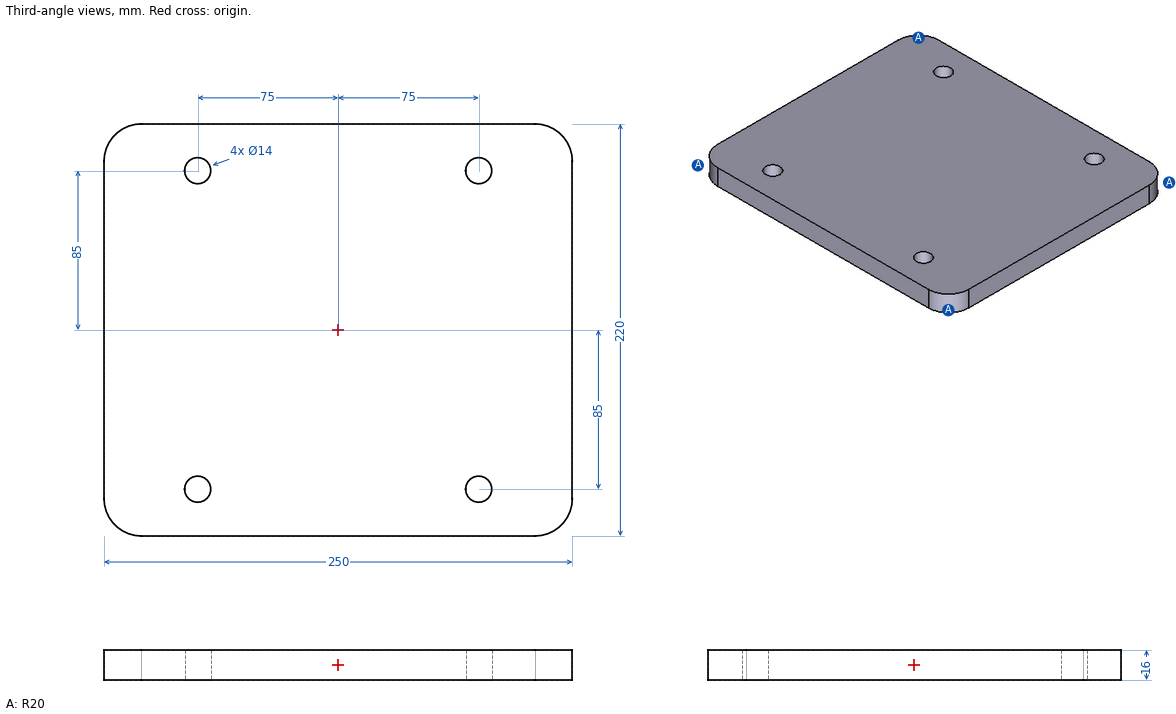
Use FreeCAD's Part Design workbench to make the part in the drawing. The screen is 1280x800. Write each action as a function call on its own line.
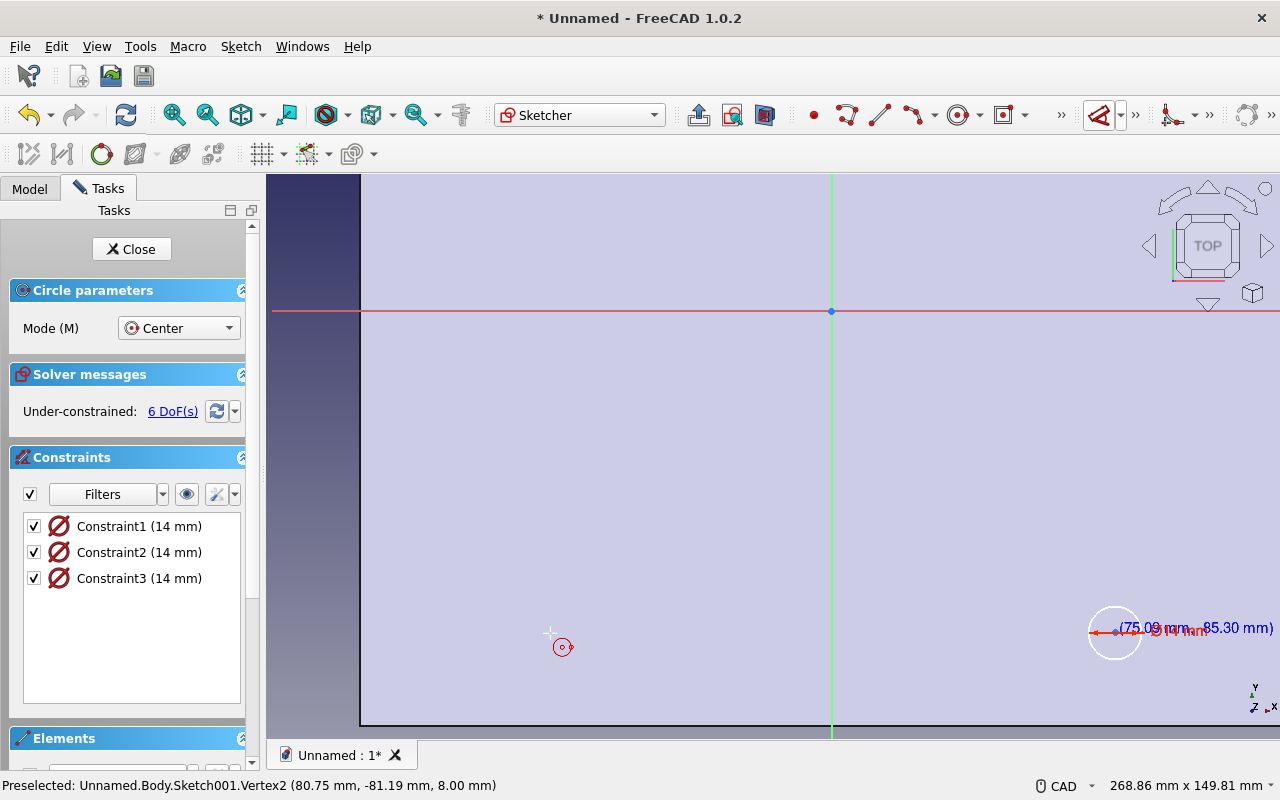
click(549, 632)
move(568, 613)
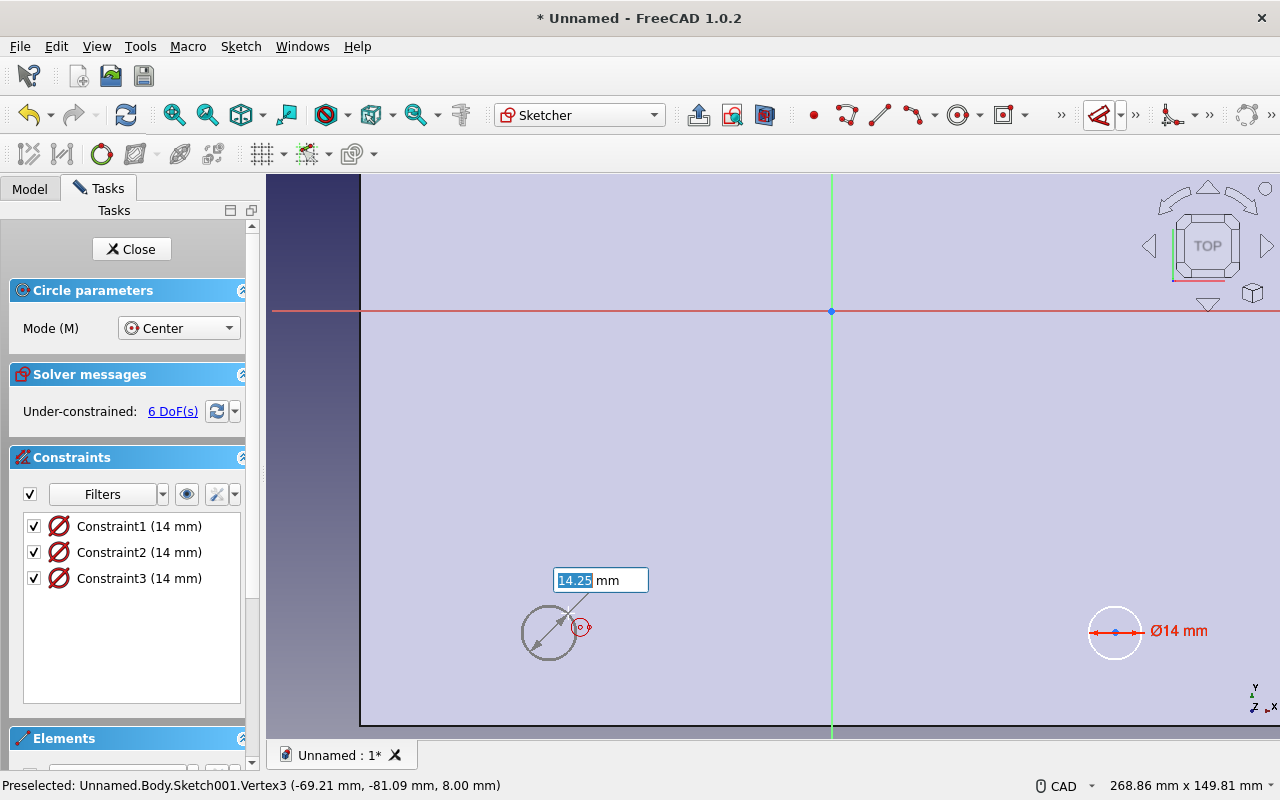
text(14)
key(Return)
key(Escape)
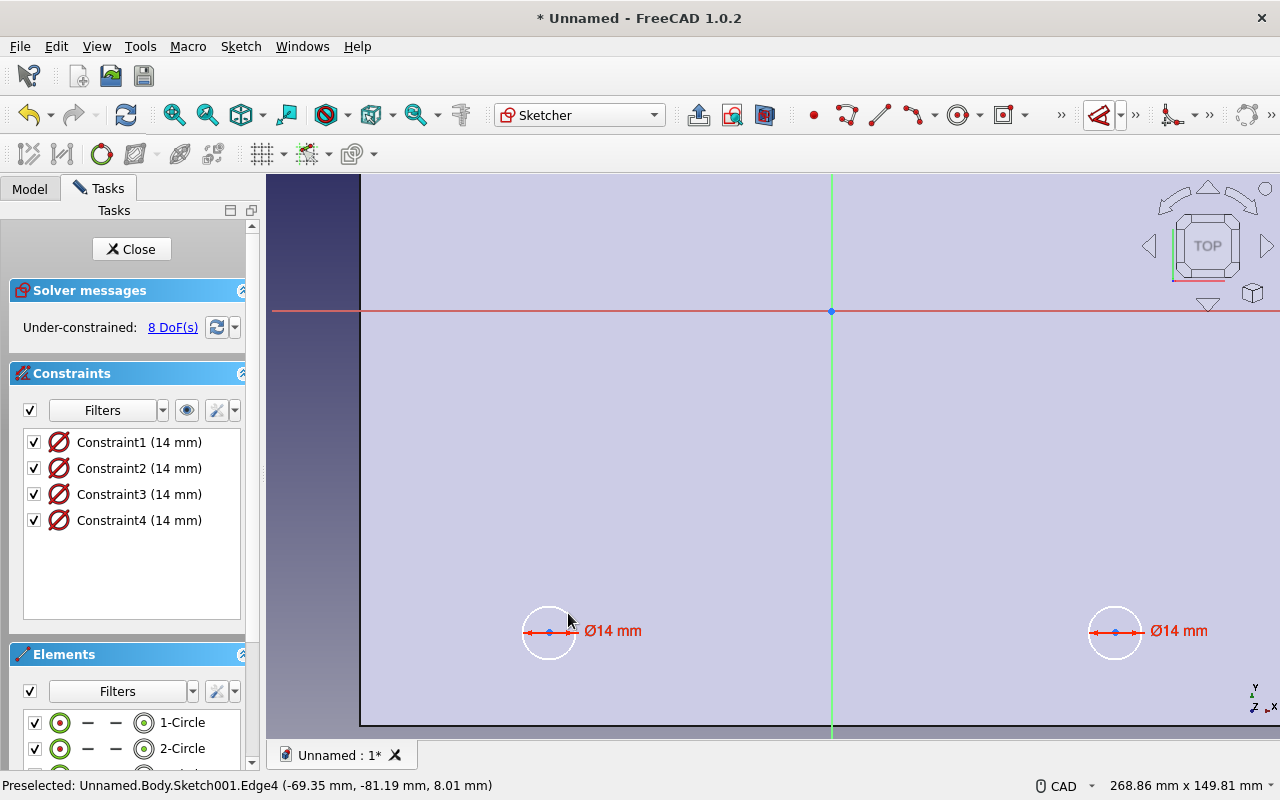
scroll(550, 633, down, 3)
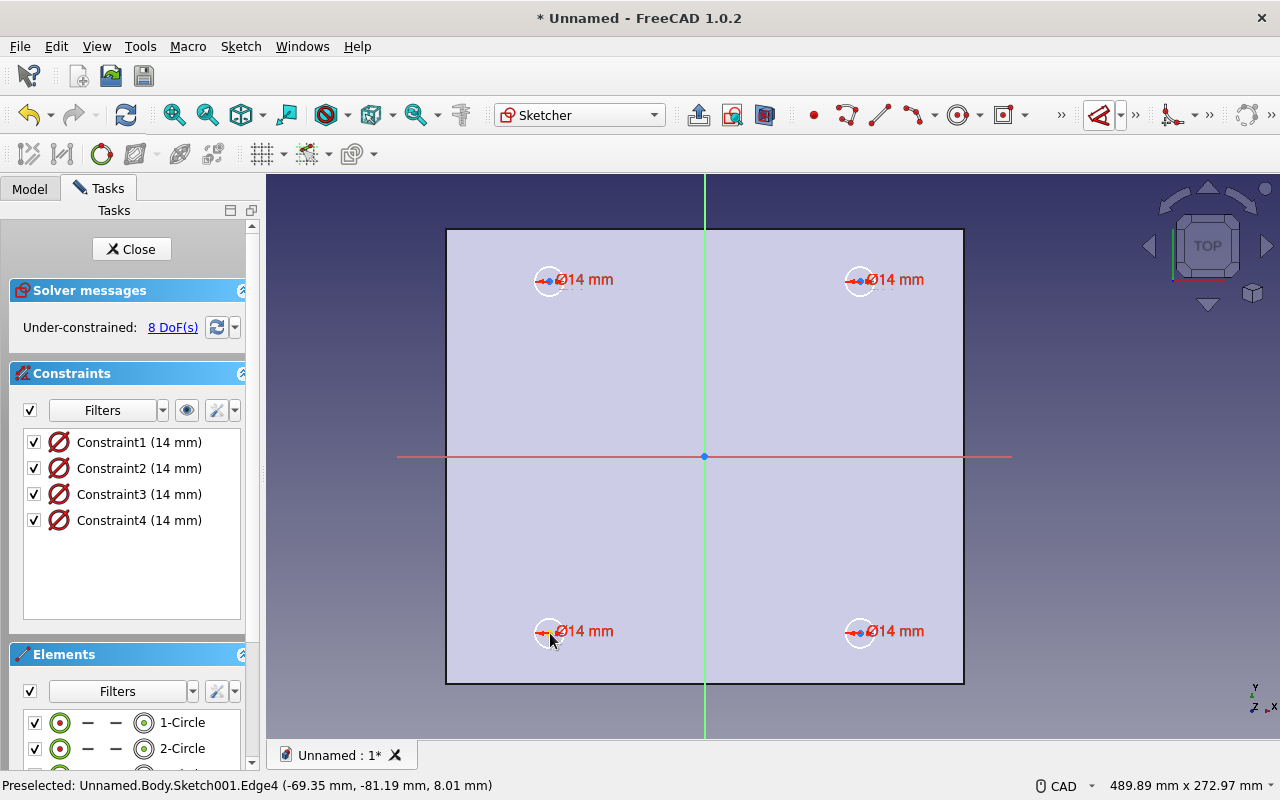
click(549, 282)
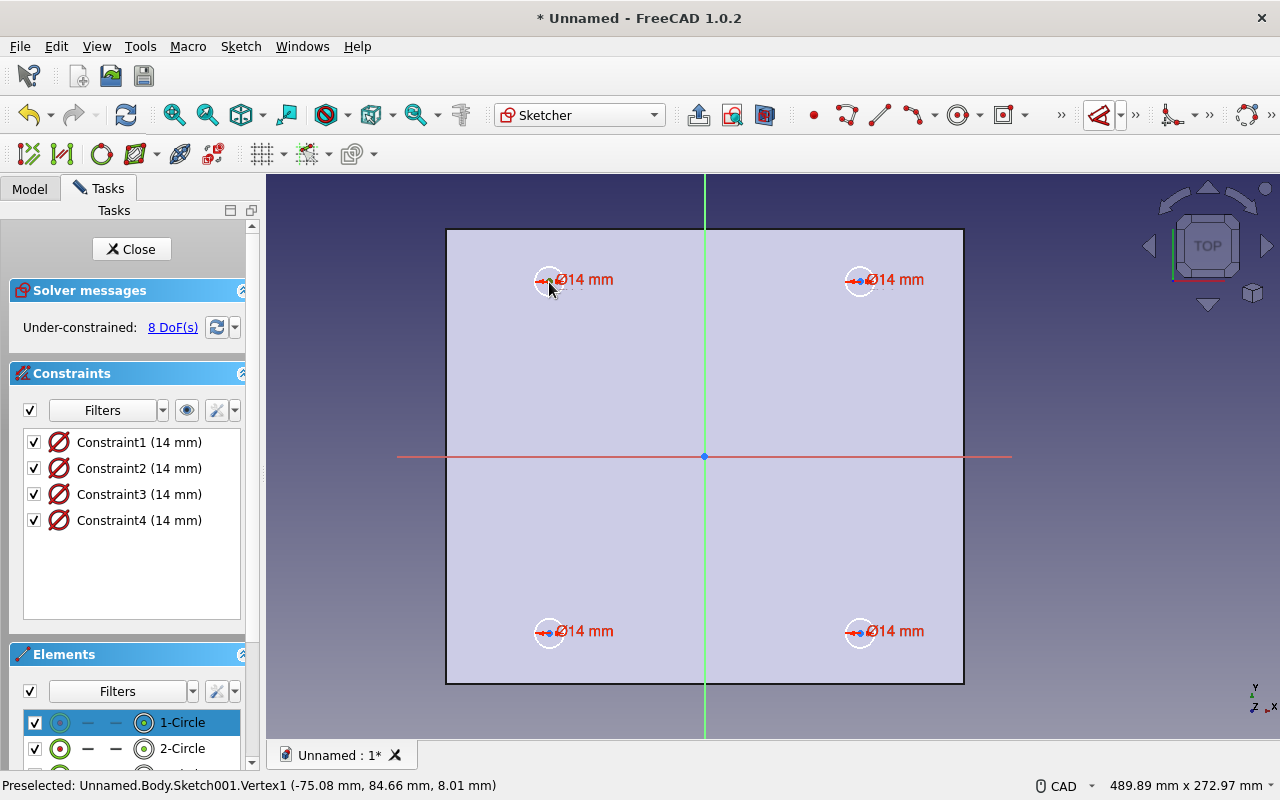
click(860, 282)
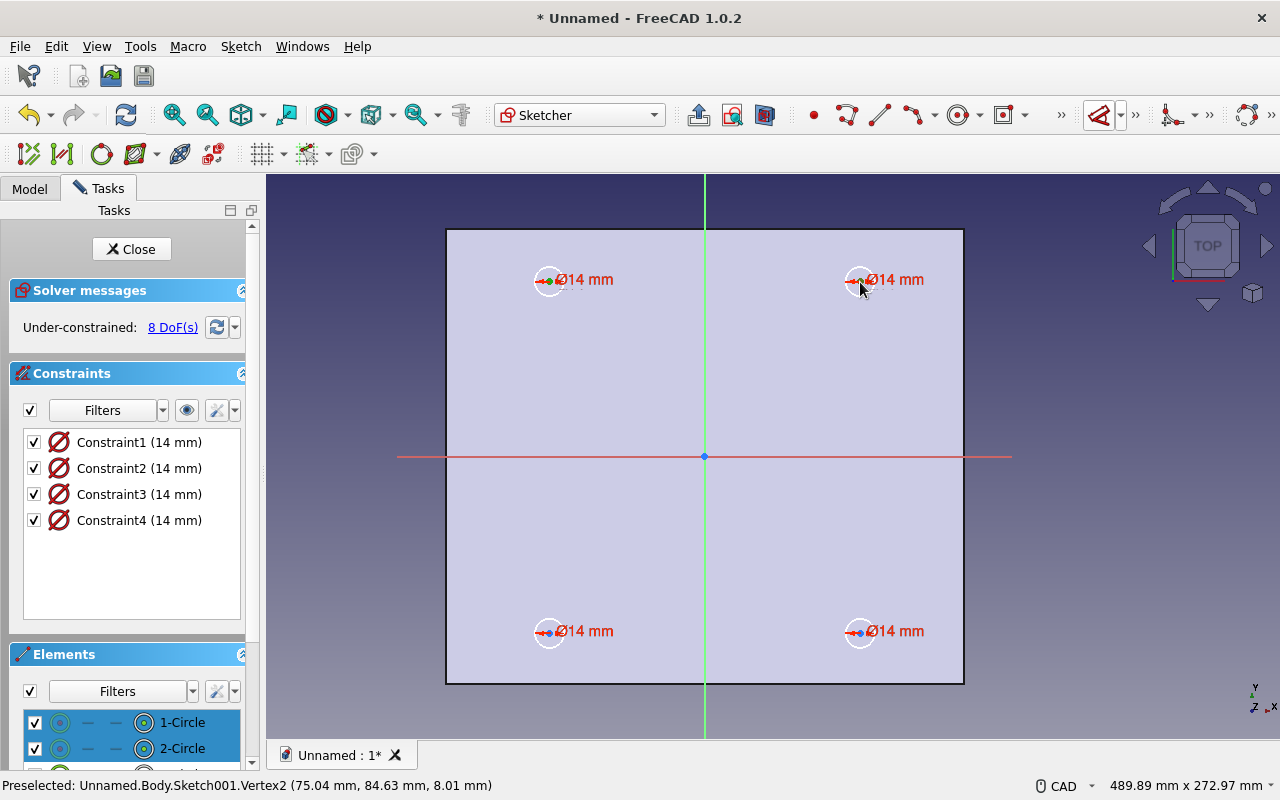
key(h)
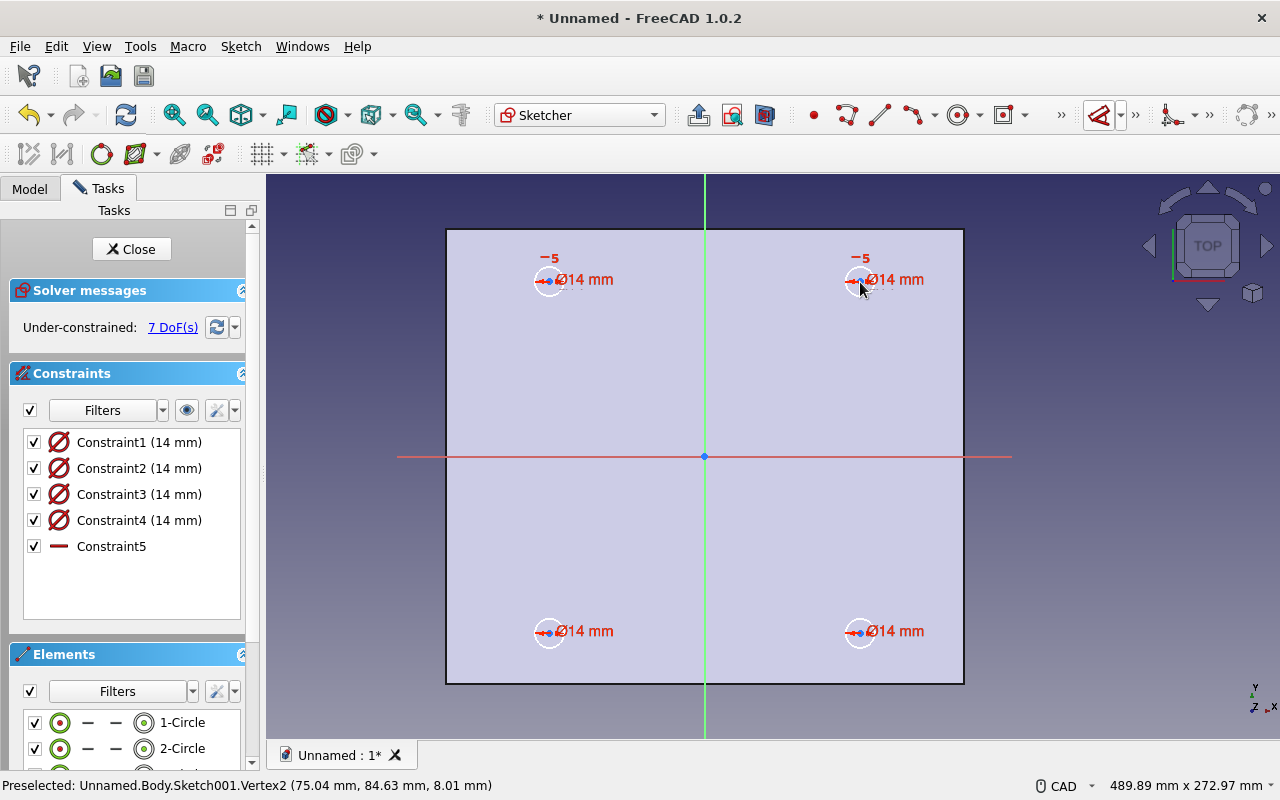
click(860, 282)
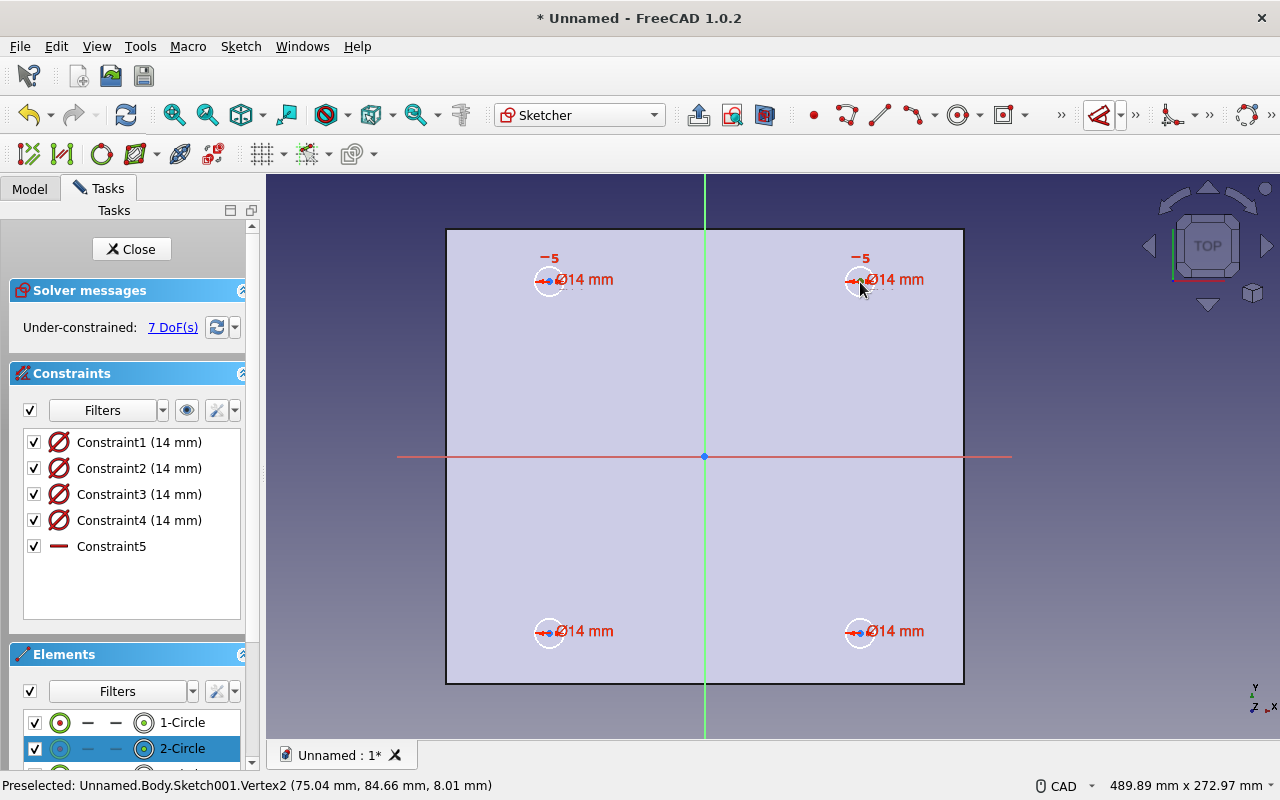
click(860, 633)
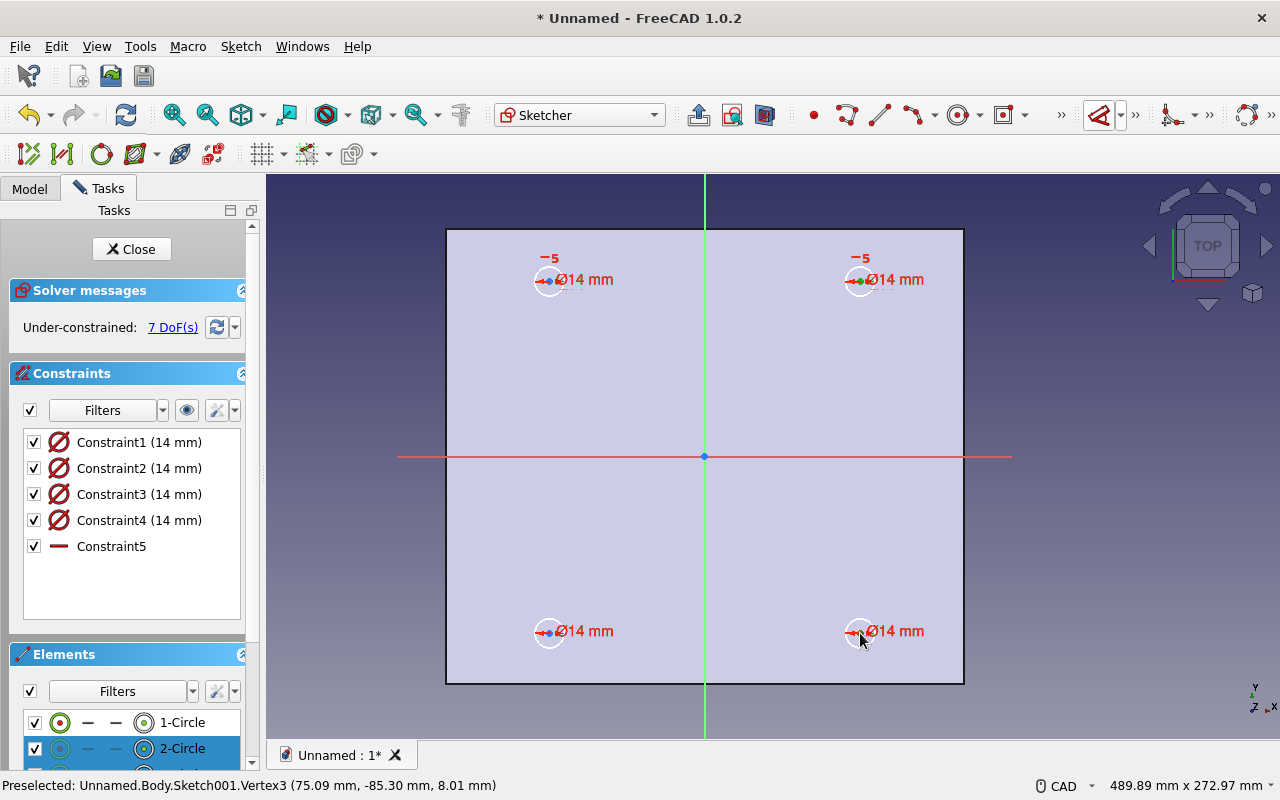
key(v)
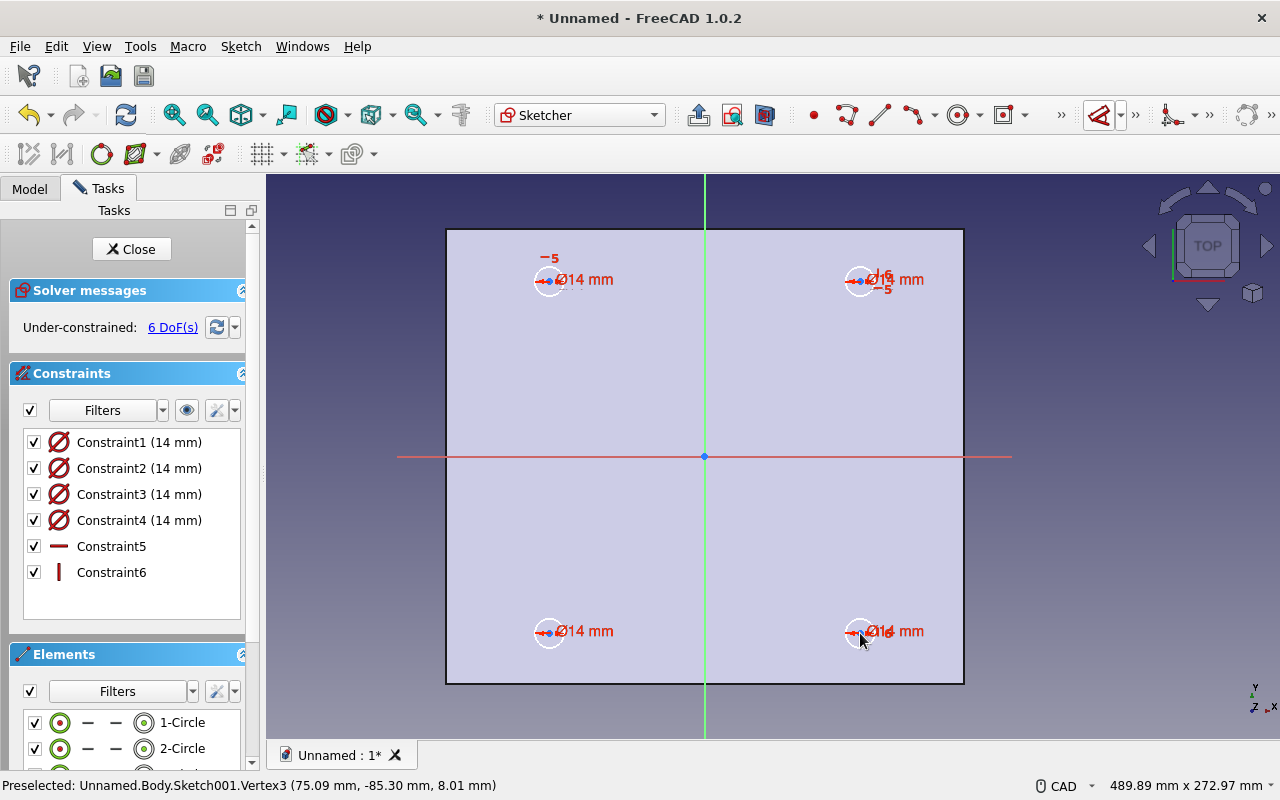
click(549, 282)